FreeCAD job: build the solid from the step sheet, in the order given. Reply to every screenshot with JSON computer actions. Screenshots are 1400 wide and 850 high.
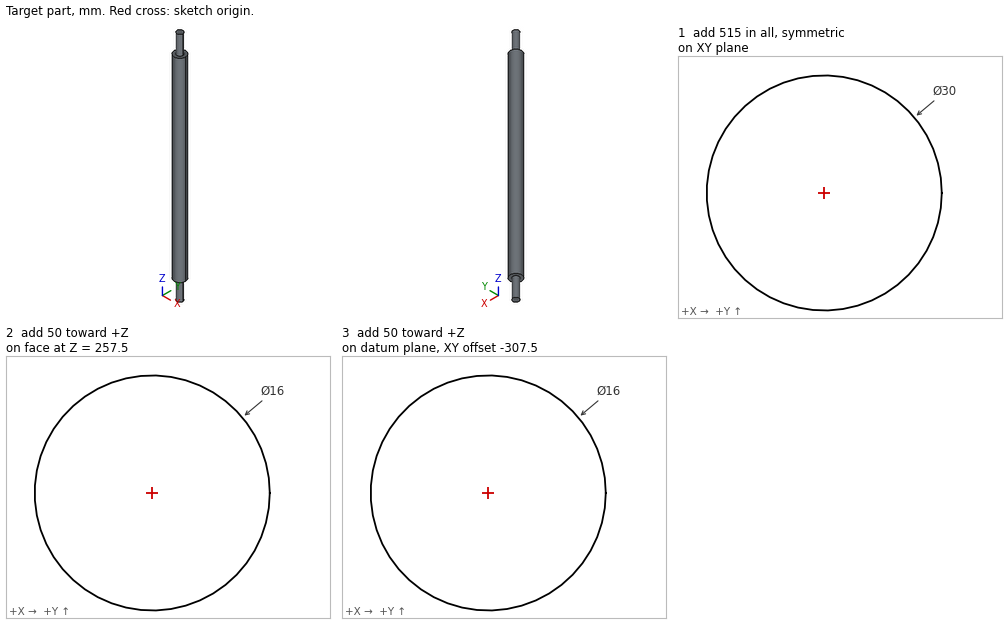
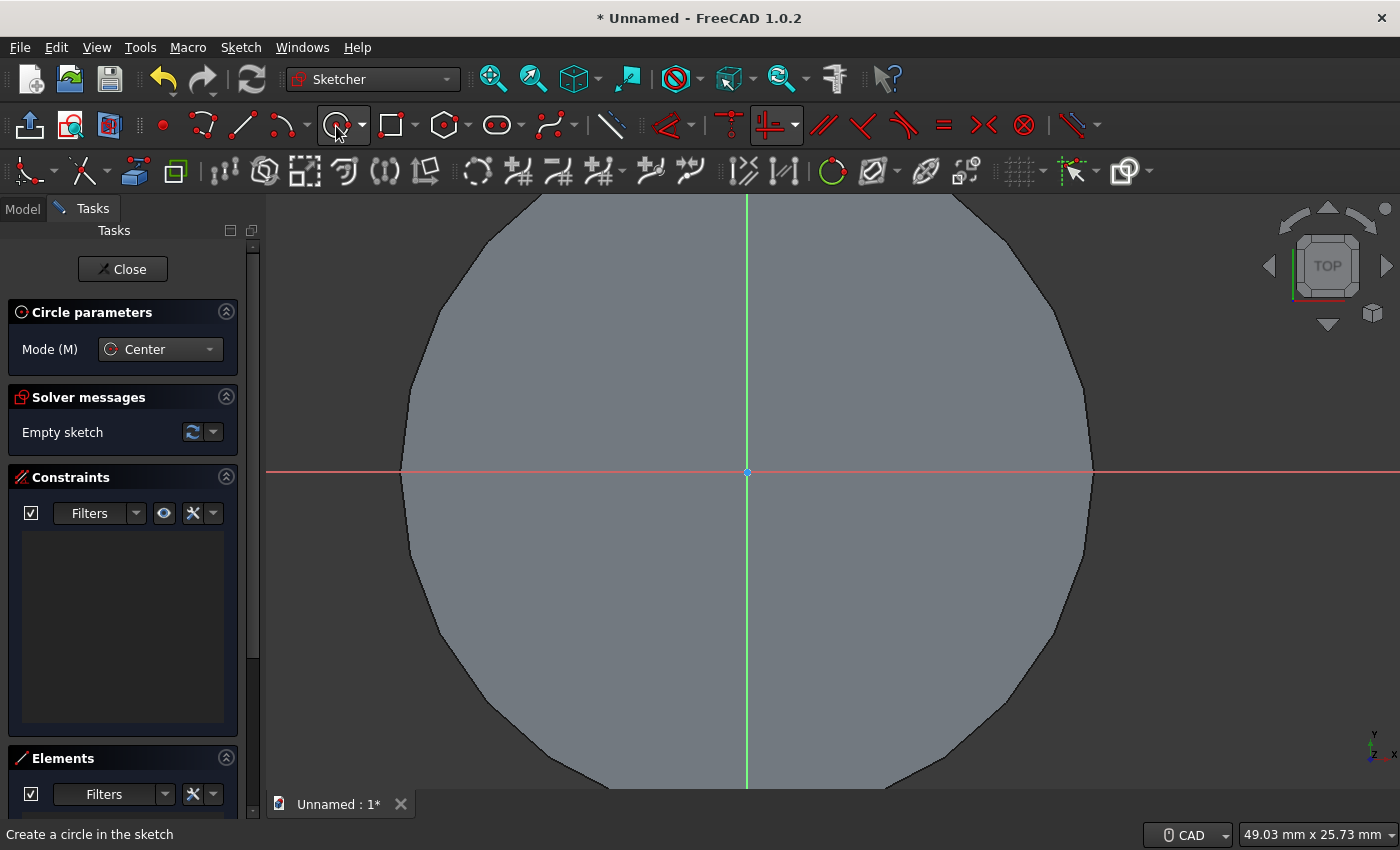
{"action": "left_click", "coordinate": [747, 472]}
{"action": "mouse_move", "coordinate": [878, 342]}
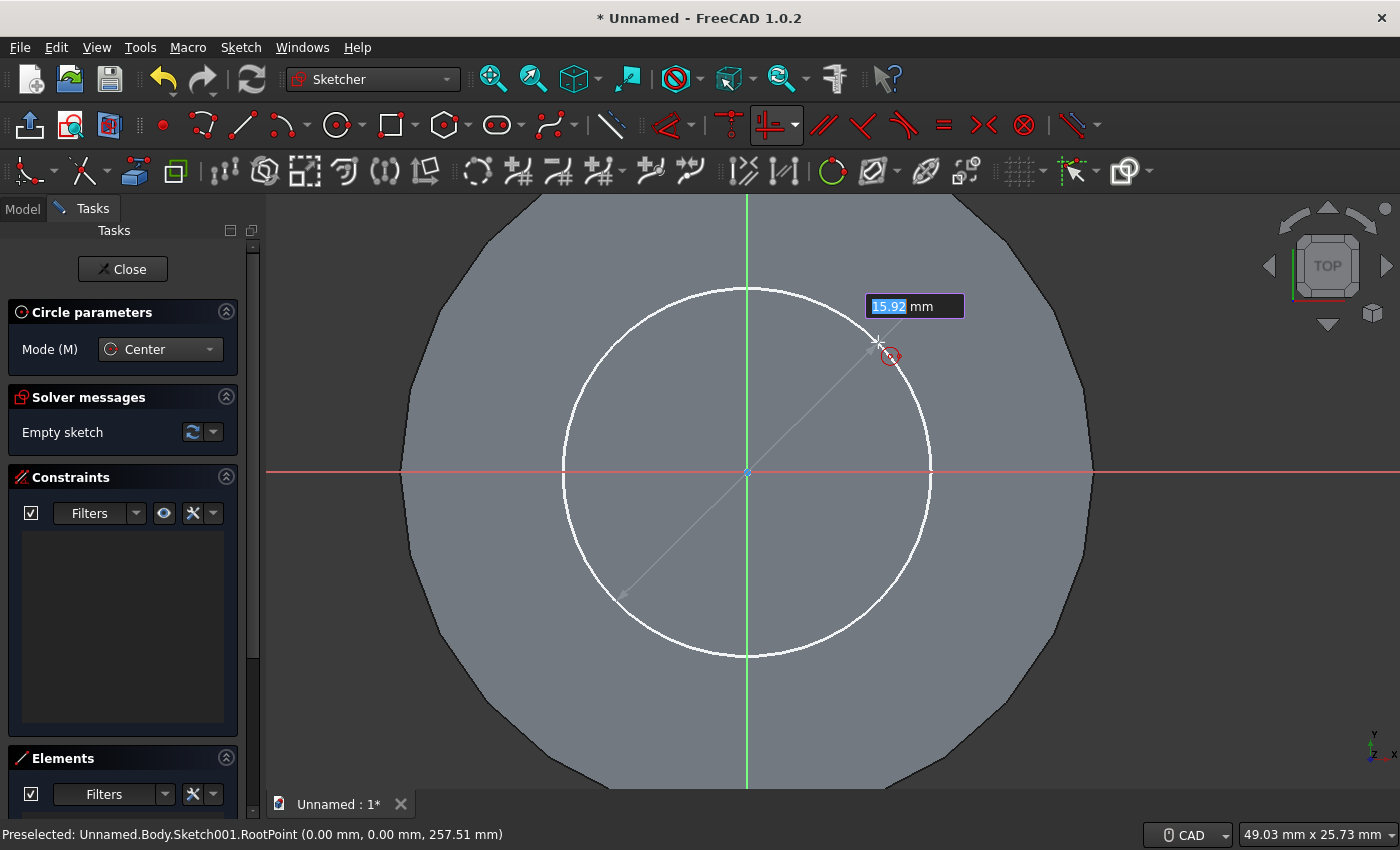
{"action": "type", "text": "16"}
{"action": "key", "text": "Return"}
{"action": "key", "text": "Escape"}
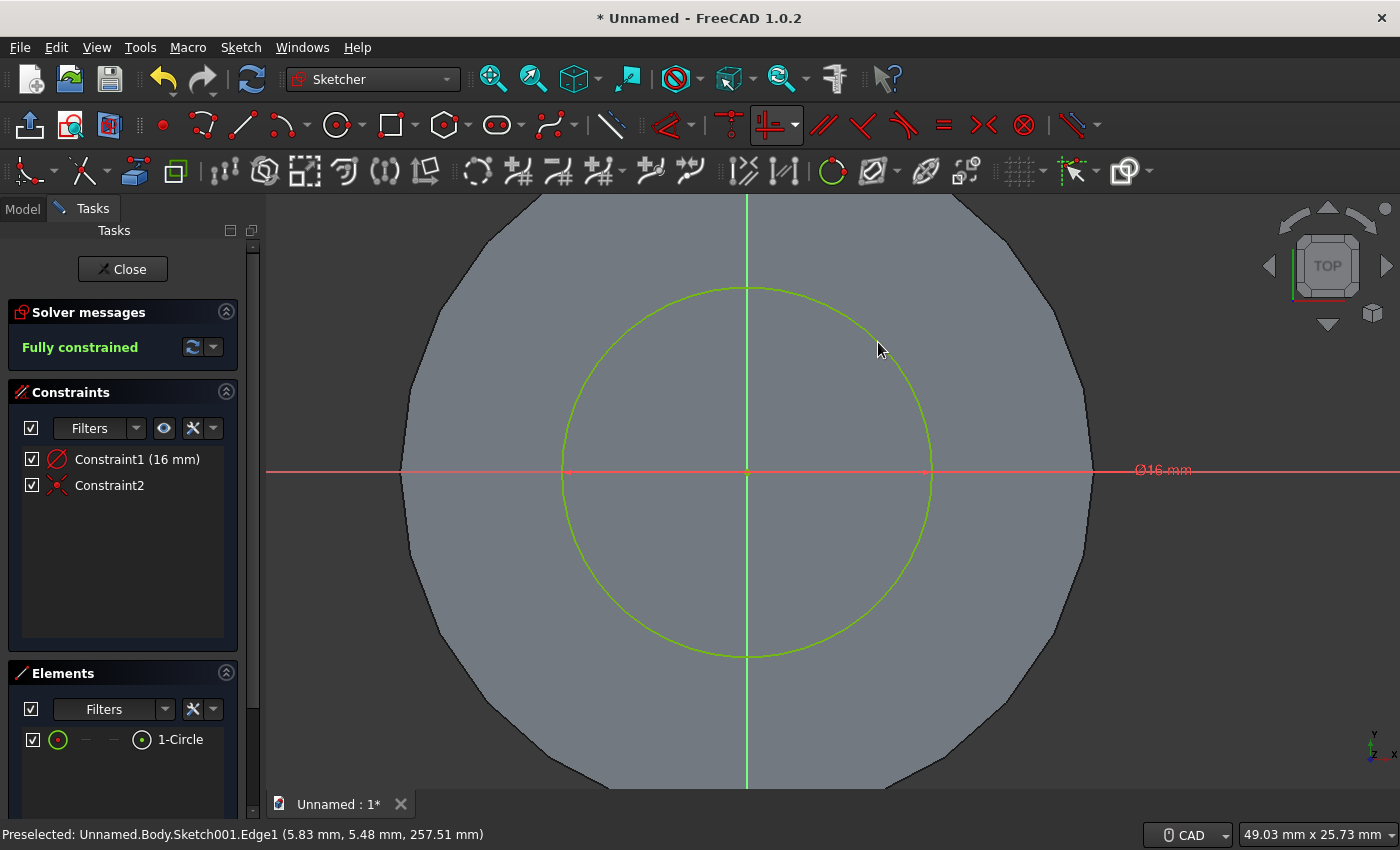
{"action": "left_click", "coordinate": [123, 269]}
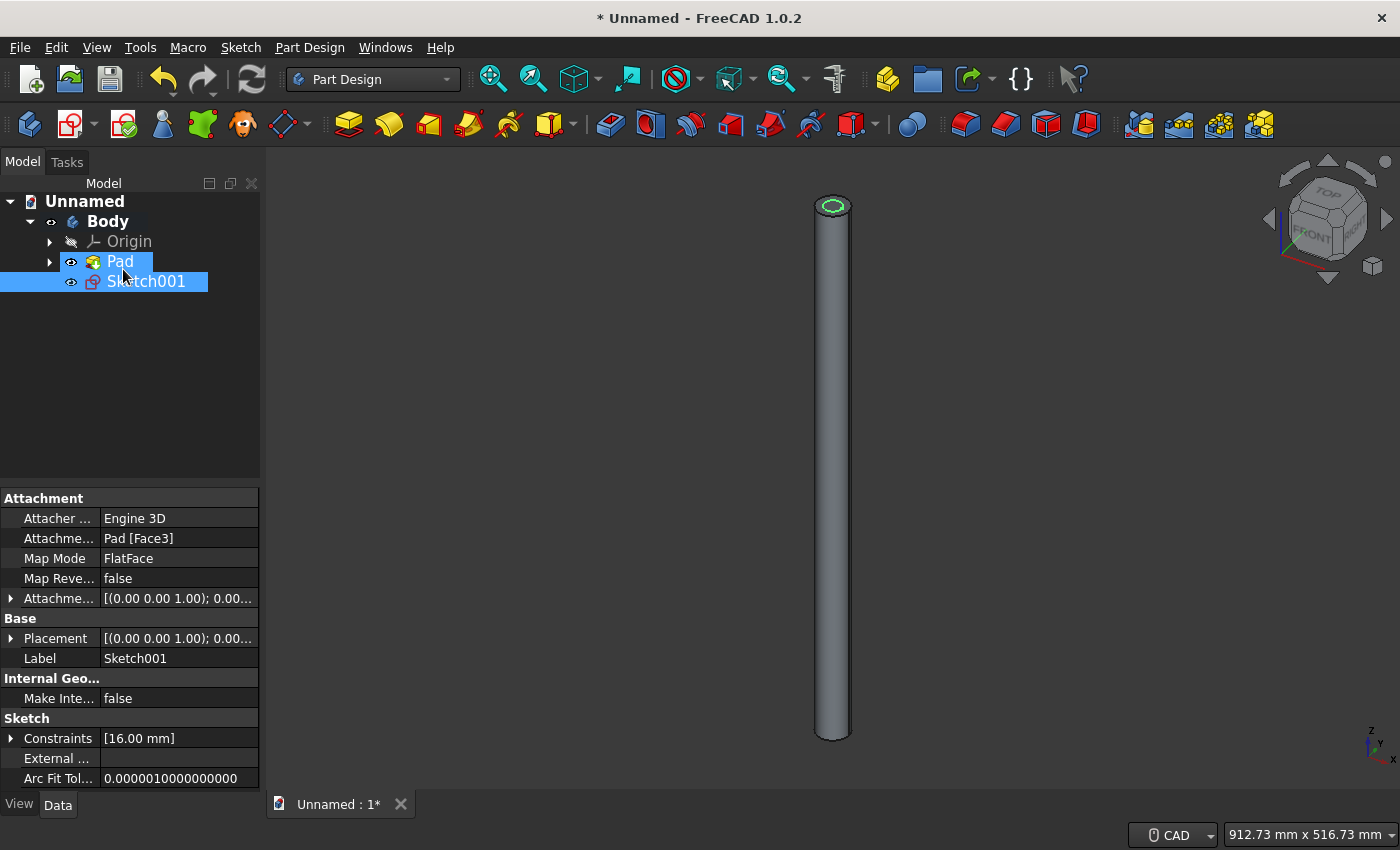
{"action": "left_click", "coordinate": [350, 124]}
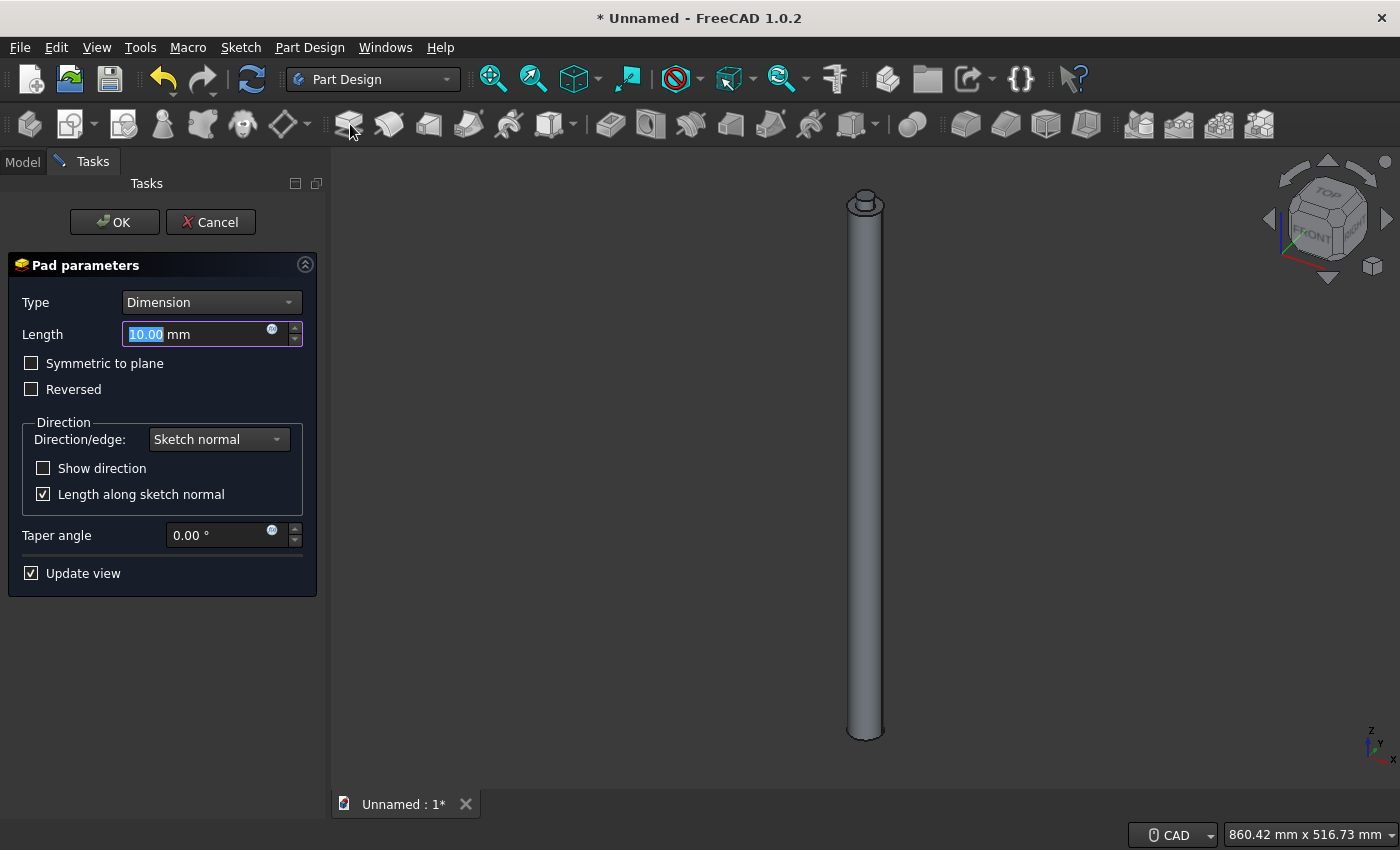
{"action": "type", "text": "50"}
{"action": "key", "text": "Tab"}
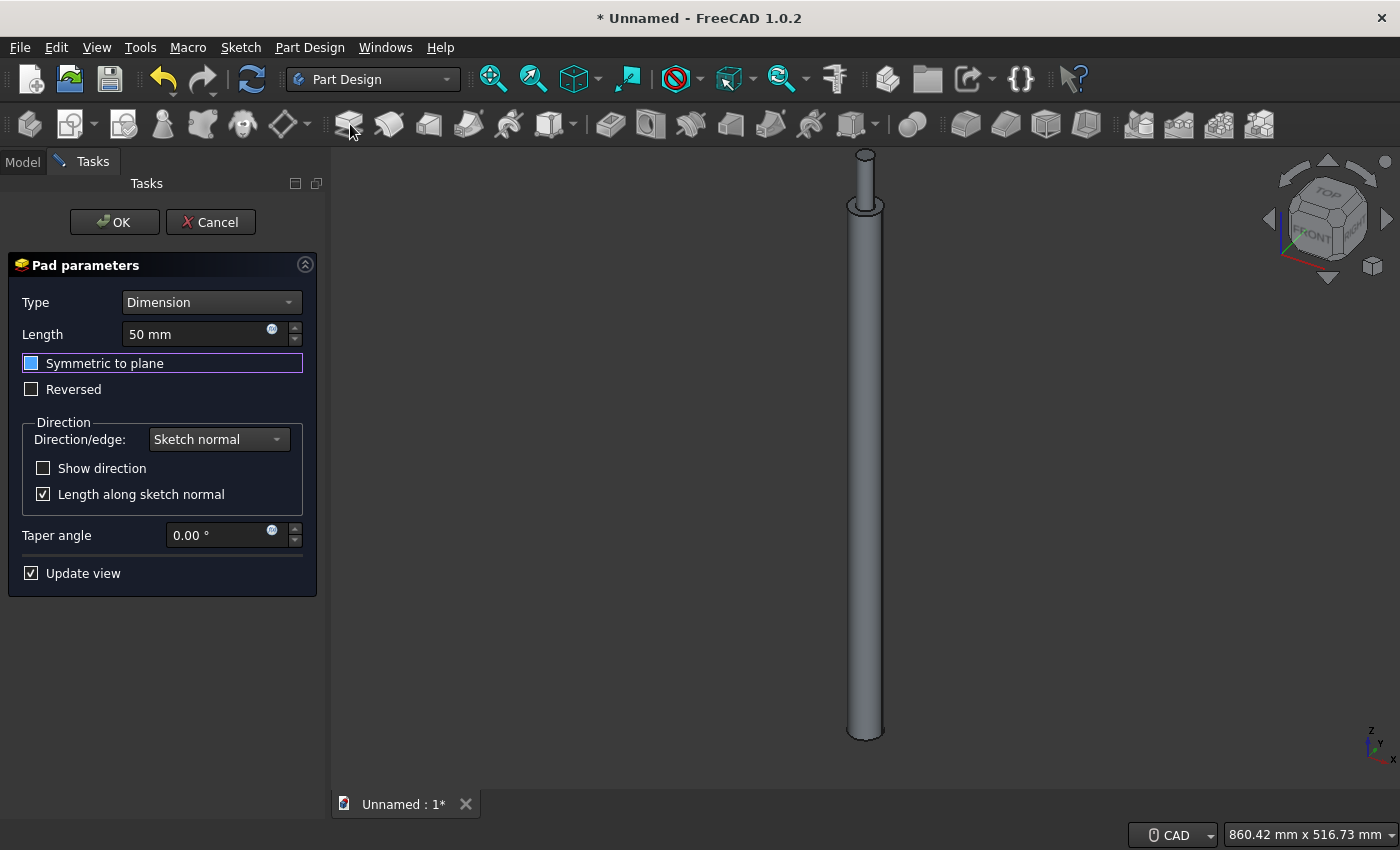
{"action": "left_click", "coordinate": [115, 222]}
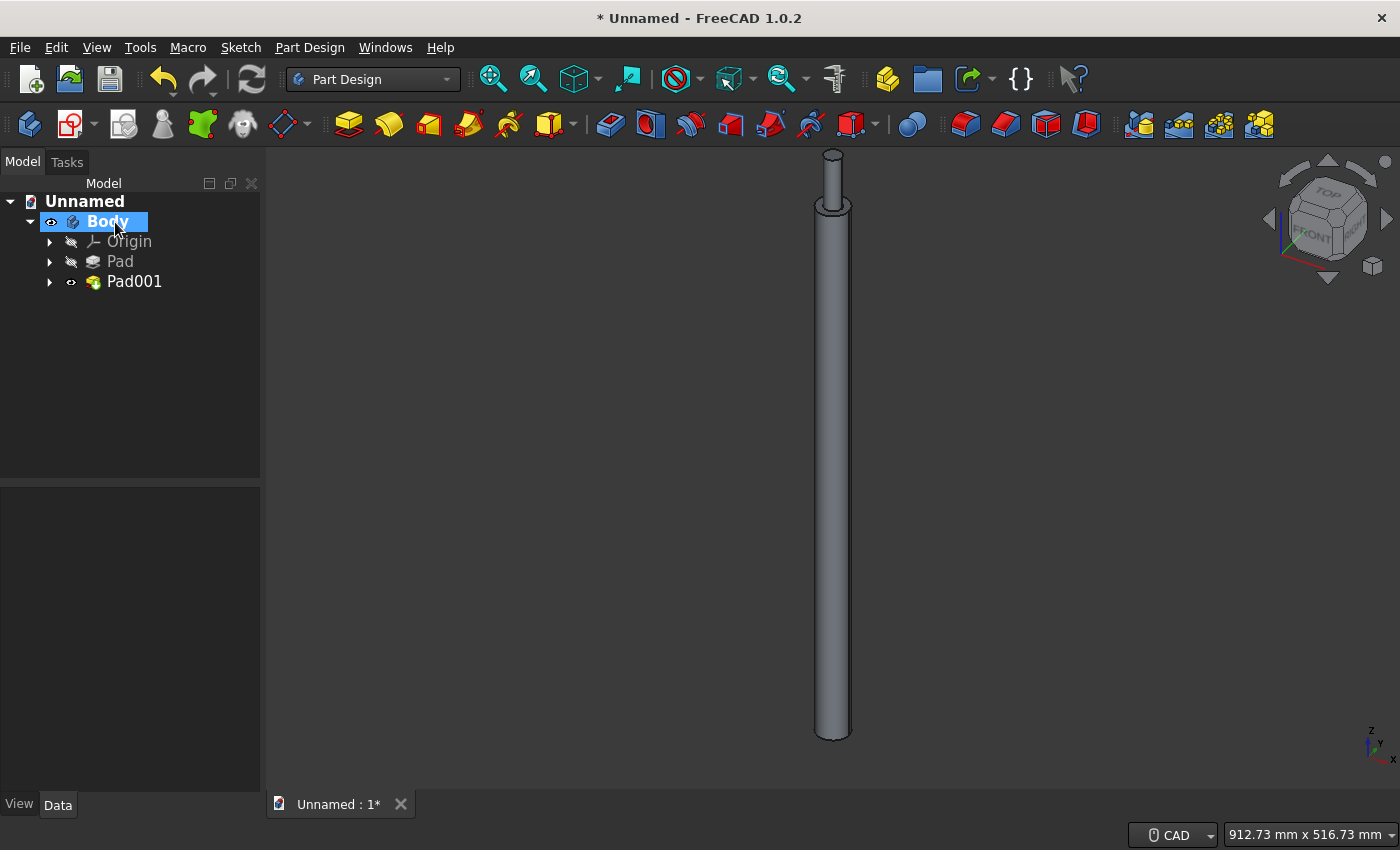
{"action": "left_click", "coordinate": [494, 80]}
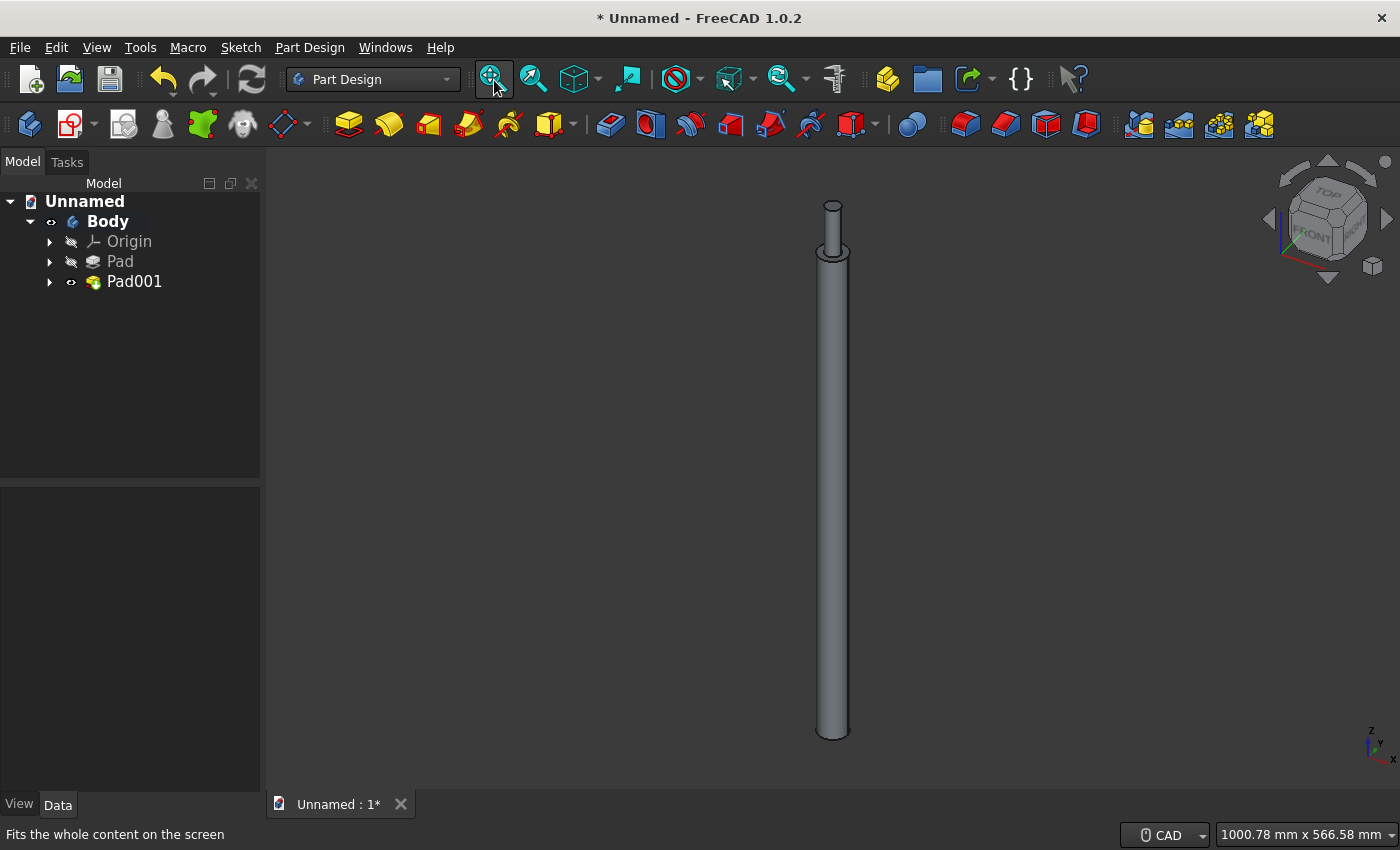
{"action": "left_click", "coordinate": [50, 242]}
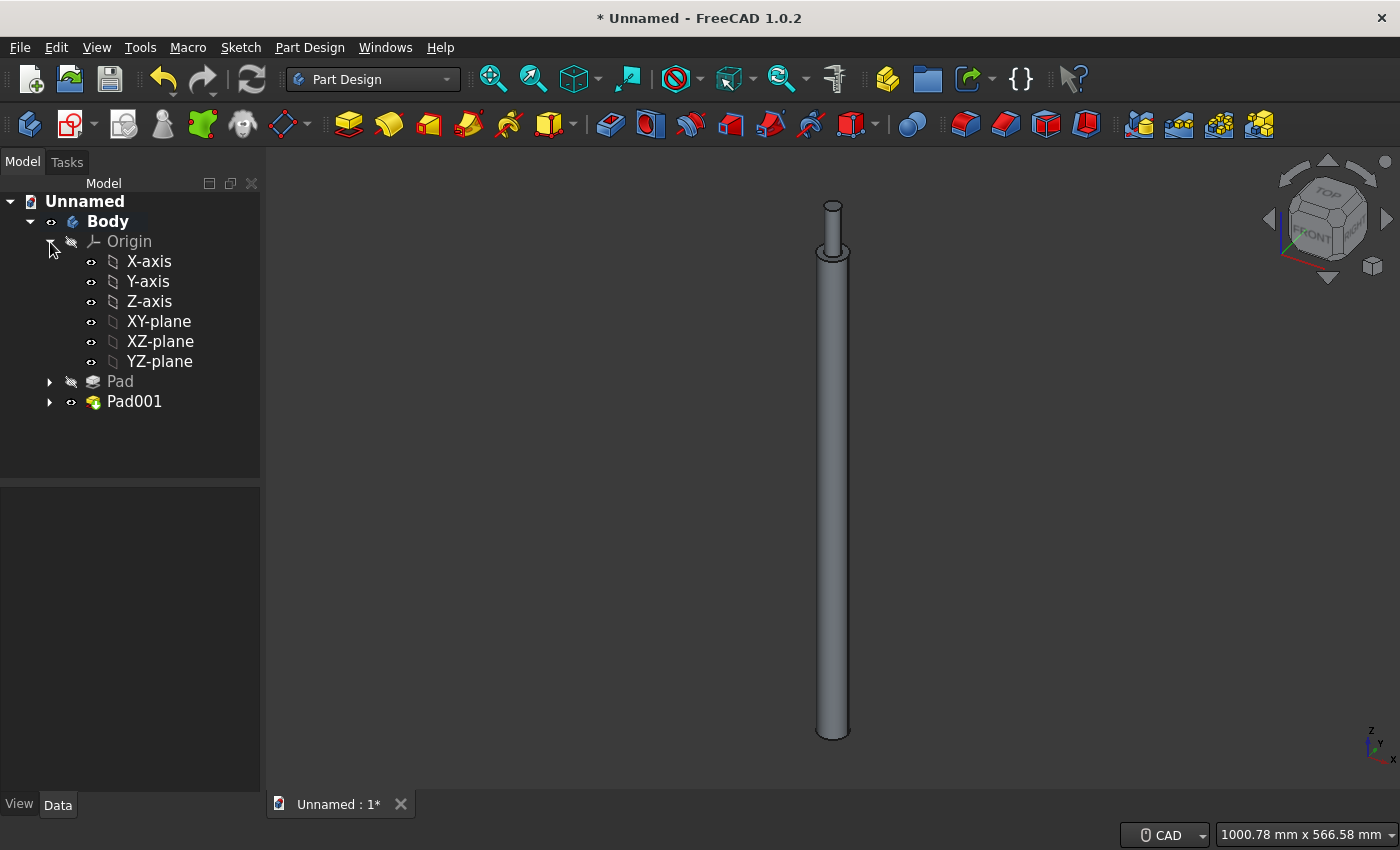
{"action": "left_click", "coordinate": [136, 322]}